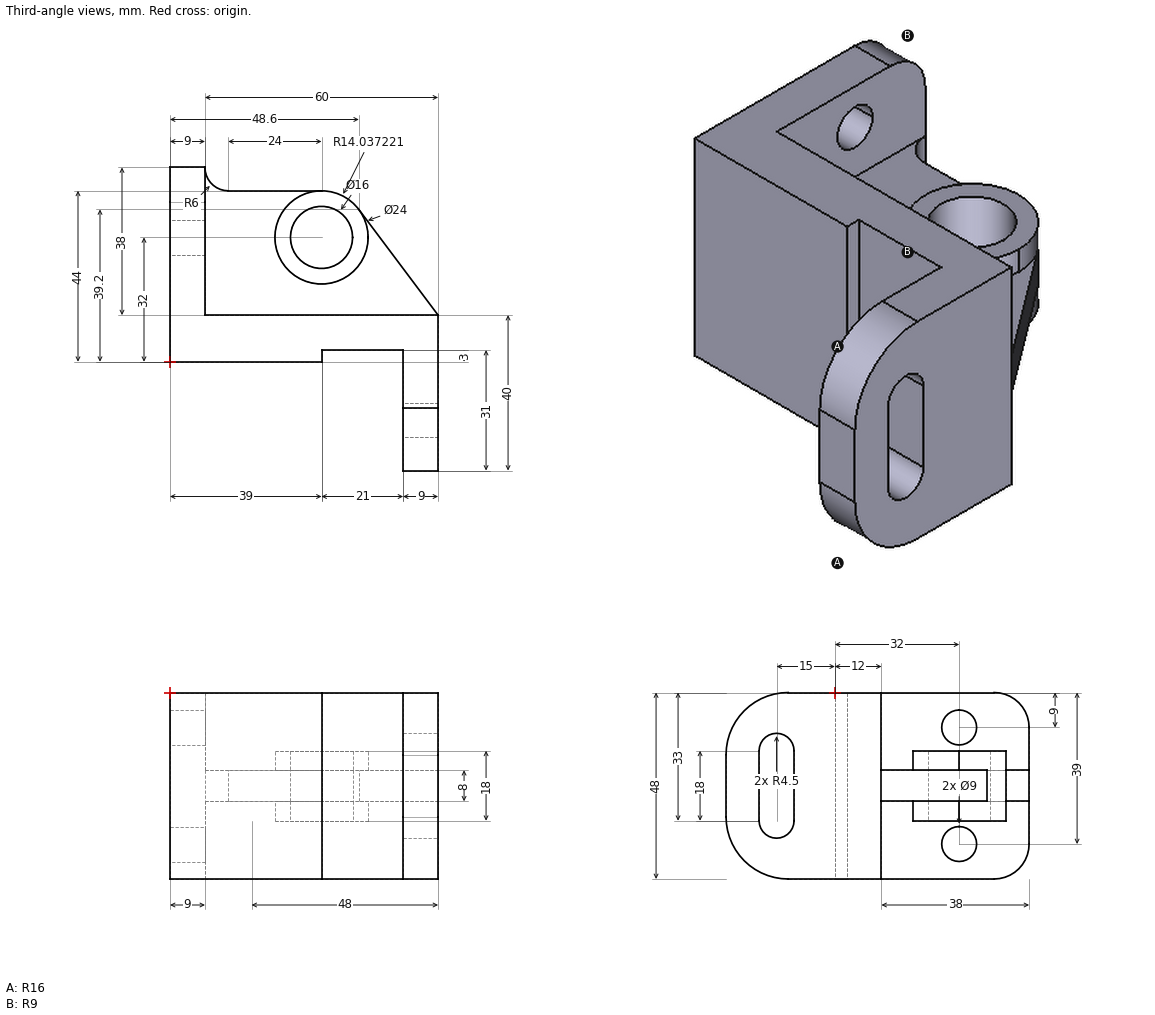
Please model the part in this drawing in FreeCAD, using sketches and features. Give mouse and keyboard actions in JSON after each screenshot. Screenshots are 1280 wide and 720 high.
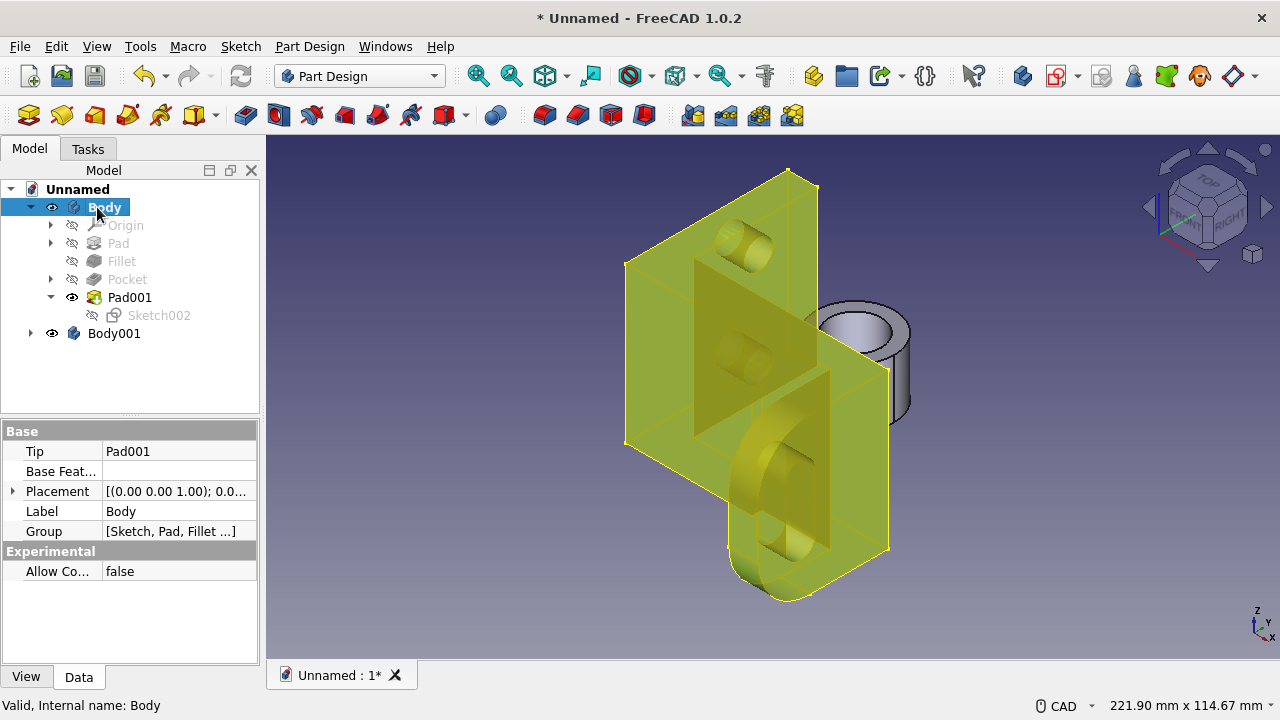
{"action": "left_click", "coordinate": [97, 207]}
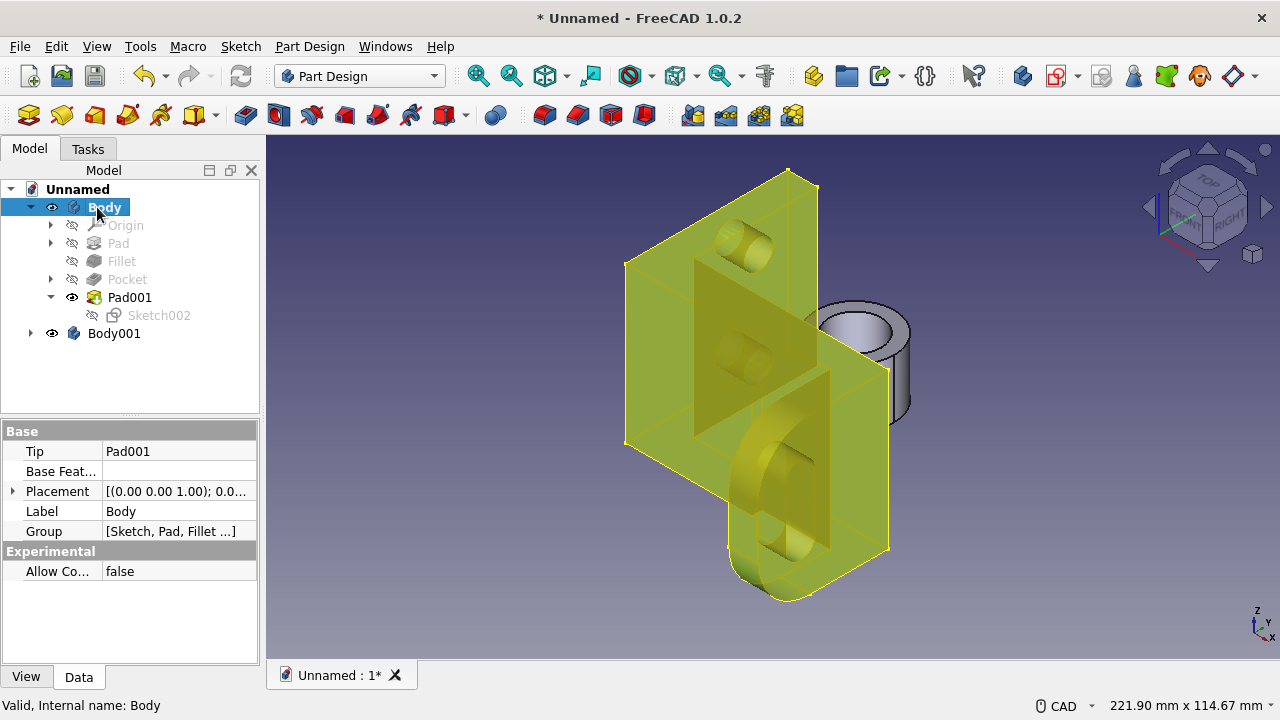
{"action": "left_click", "coordinate": [148, 571]}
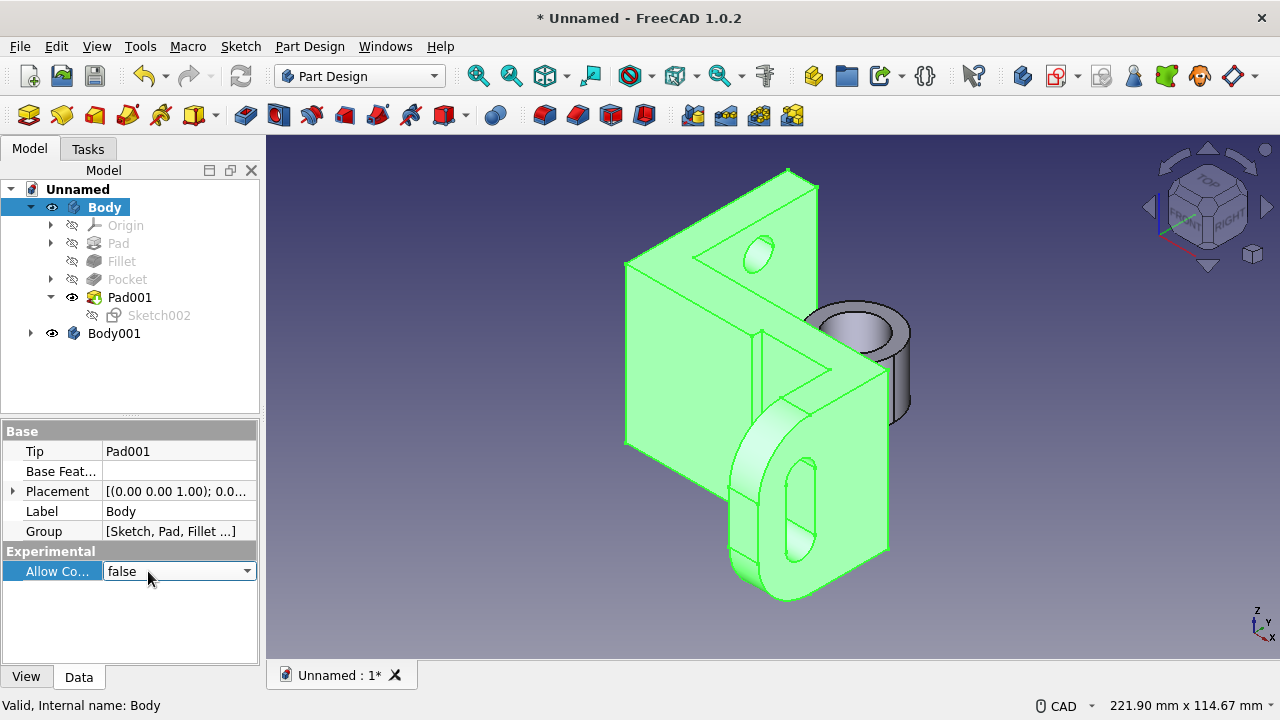
{"action": "left_click", "coordinate": [148, 571]}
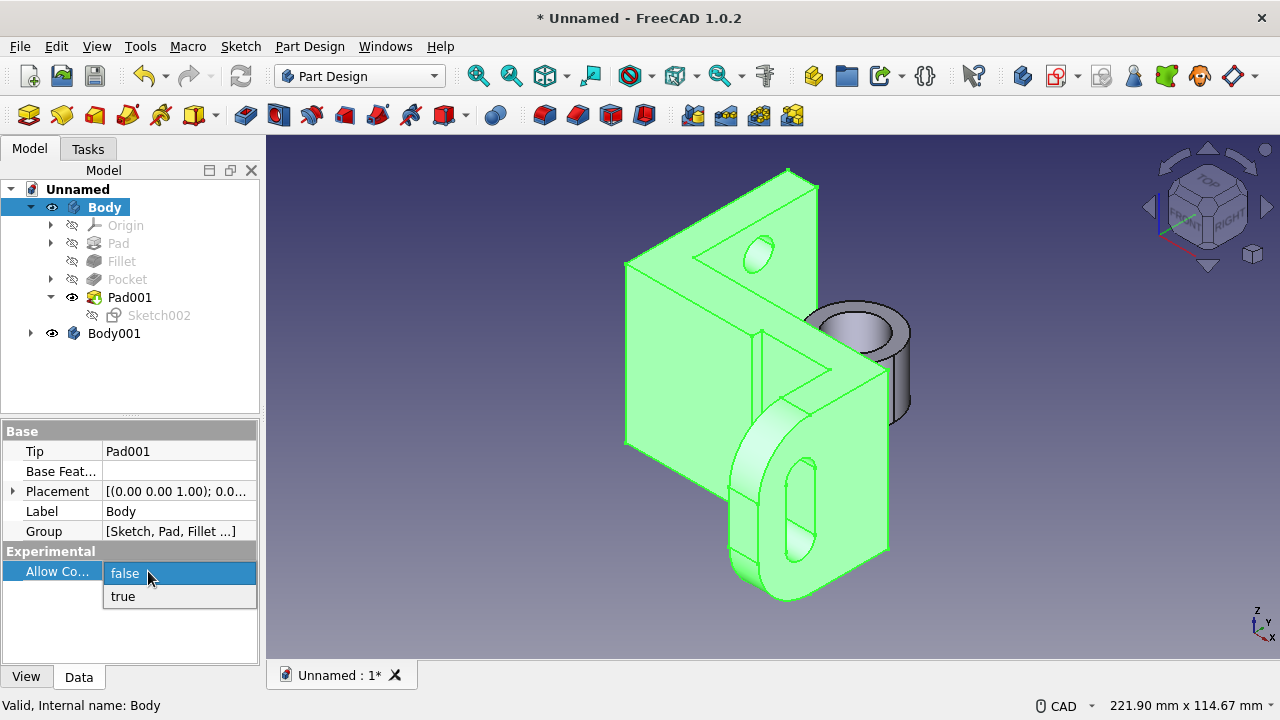
{"action": "left_click", "coordinate": [178, 596]}
{"action": "key", "text": "Return"}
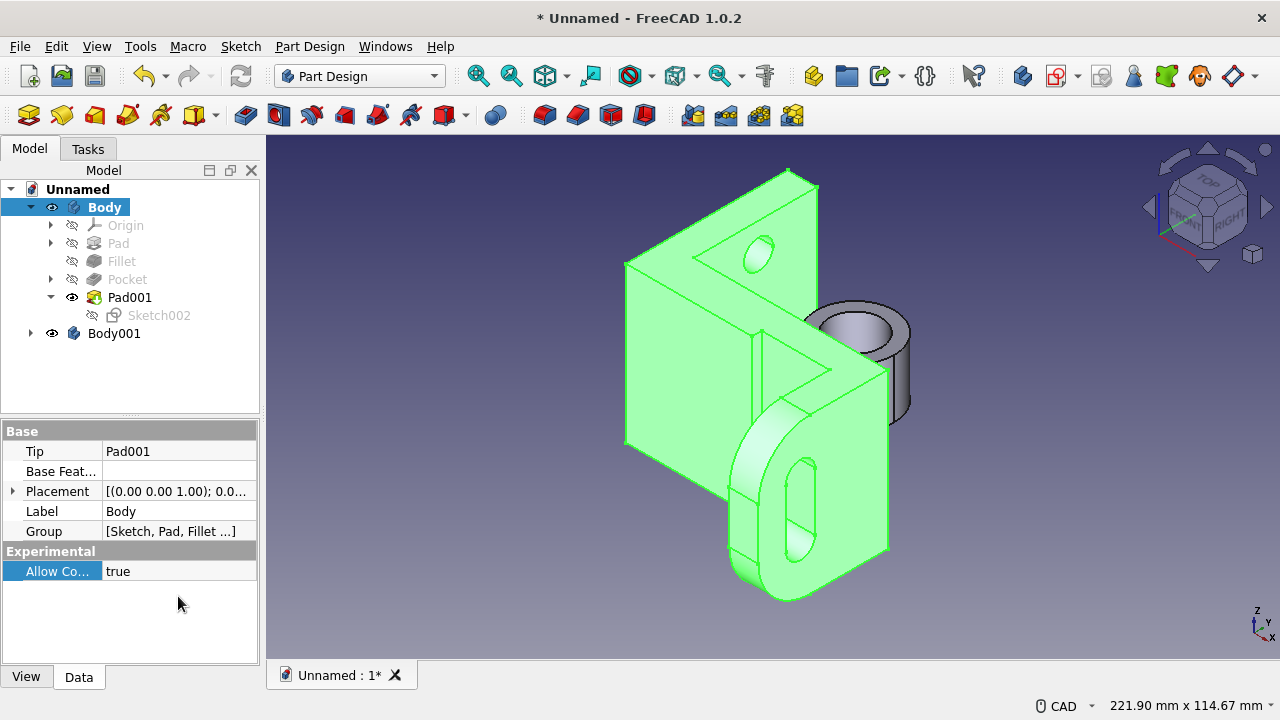
{"action": "left_click", "coordinate": [97, 333]}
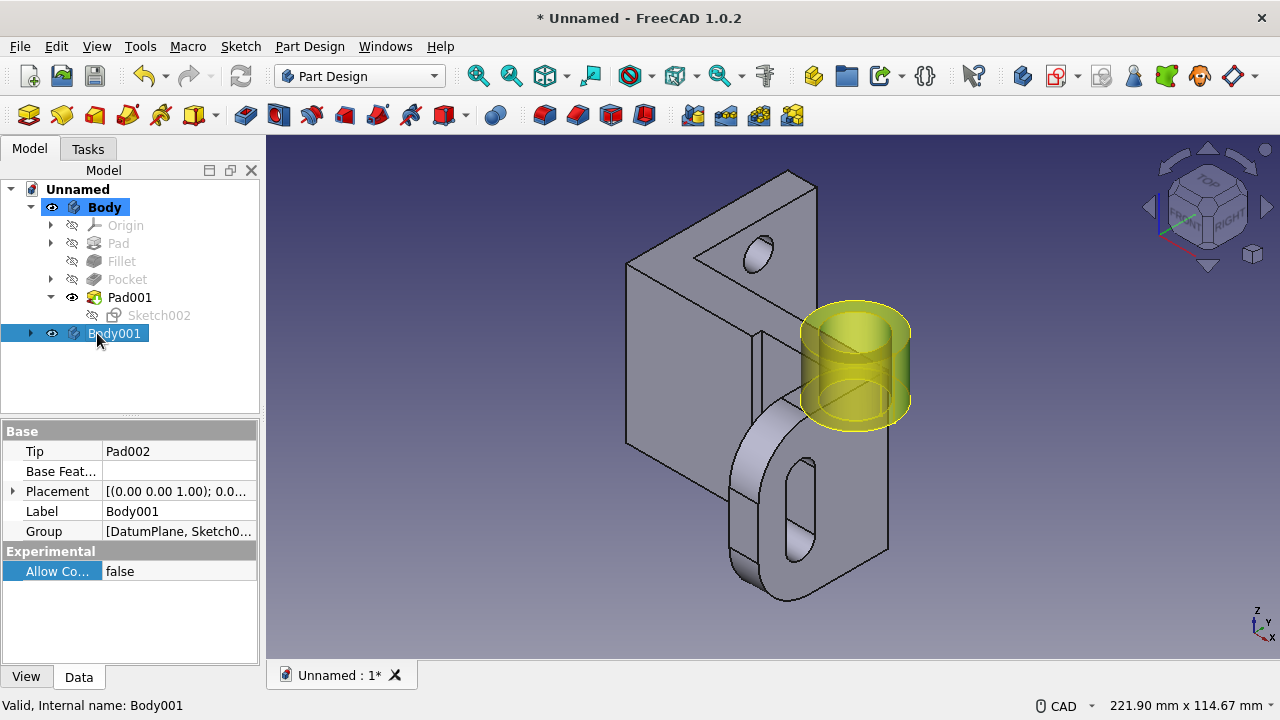
{"action": "left_click", "coordinate": [496, 116]}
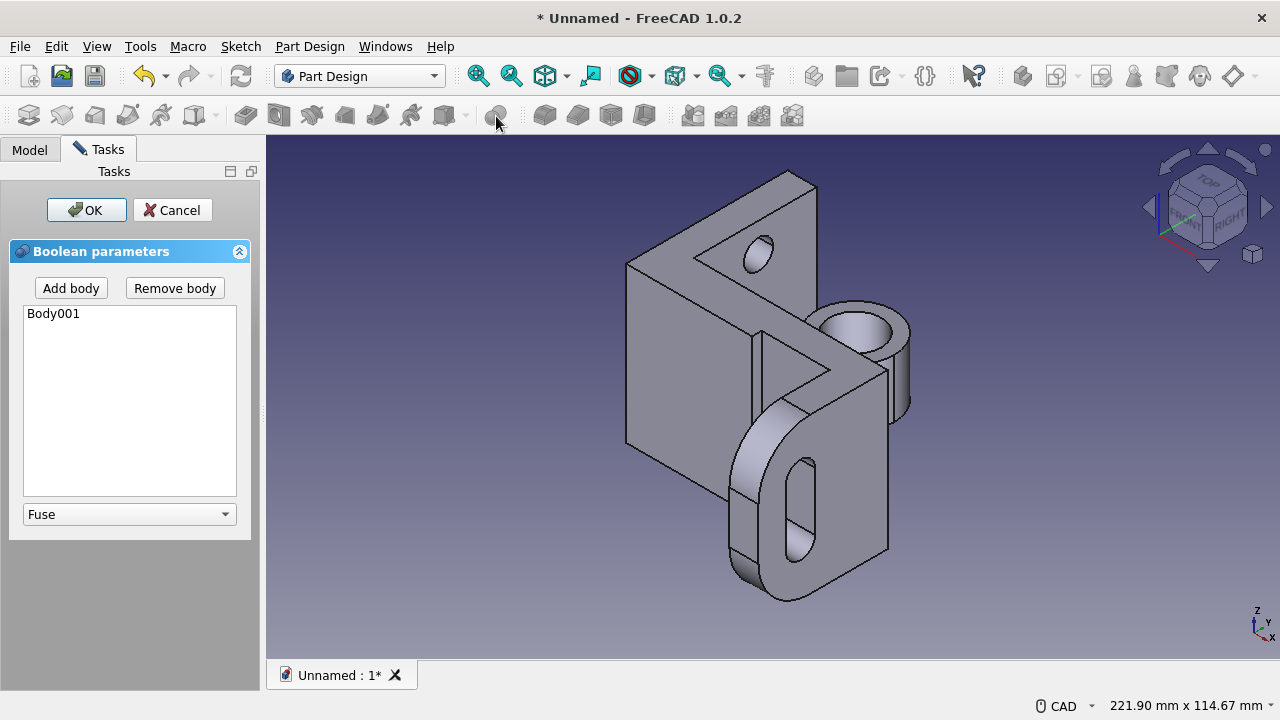
{"action": "left_click", "coordinate": [87, 210]}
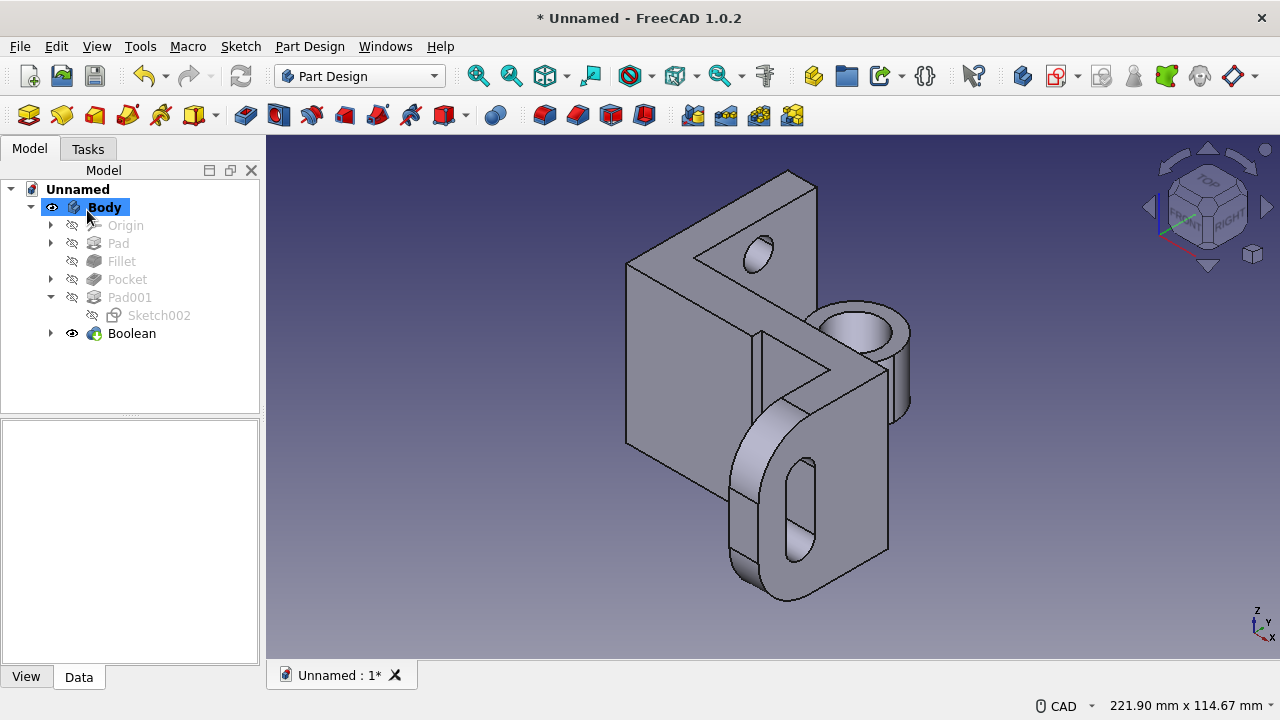
{"action": "left_click", "coordinate": [51, 225]}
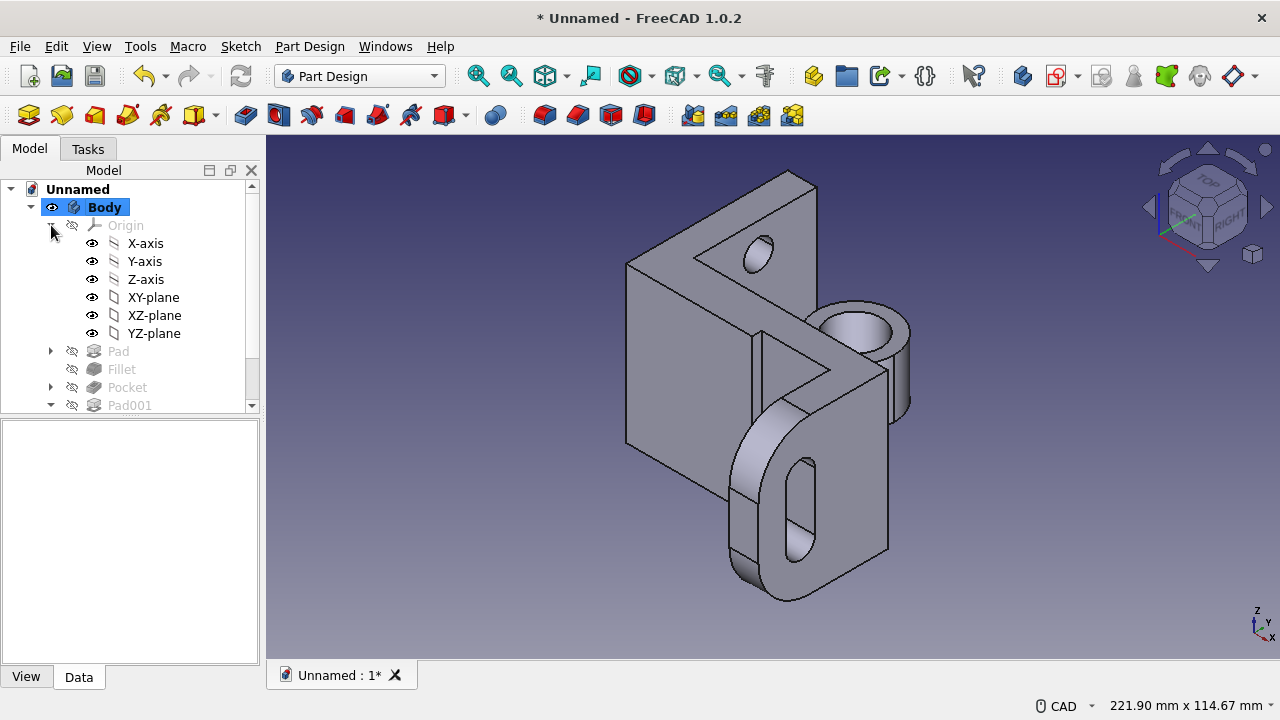
{"action": "left_click", "coordinate": [137, 297]}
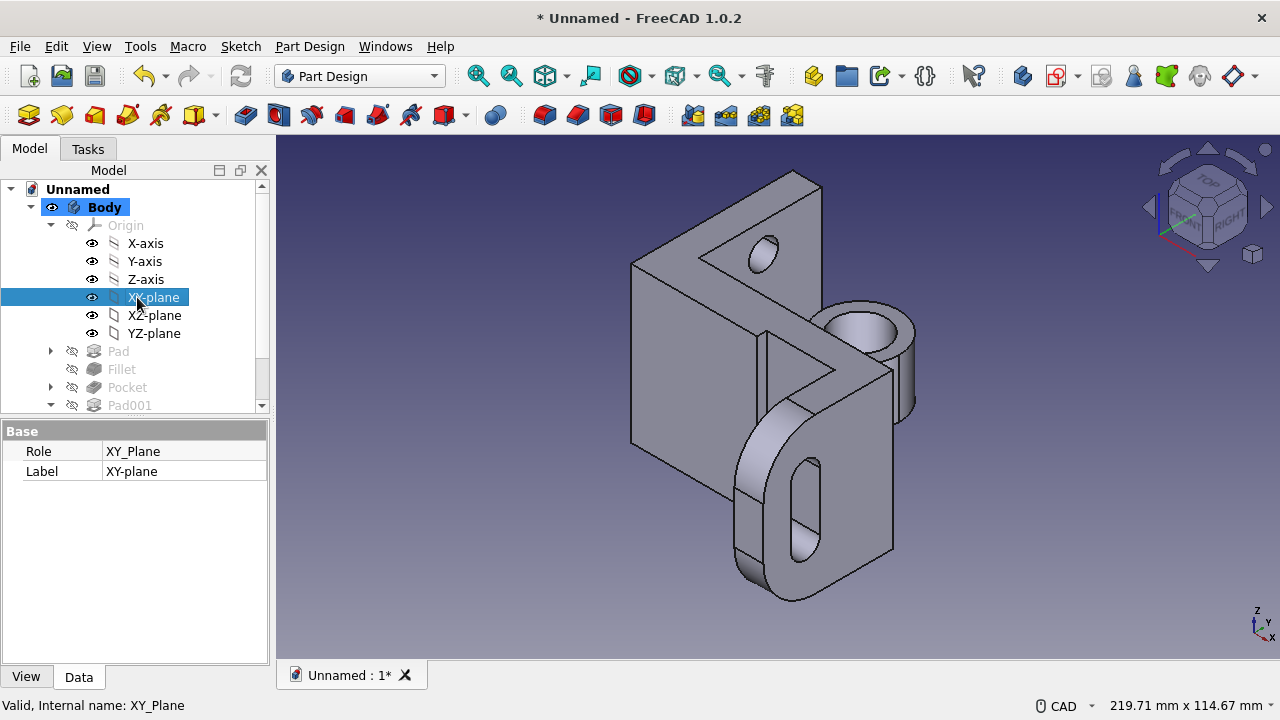
{"action": "left_click", "coordinate": [1232, 76]}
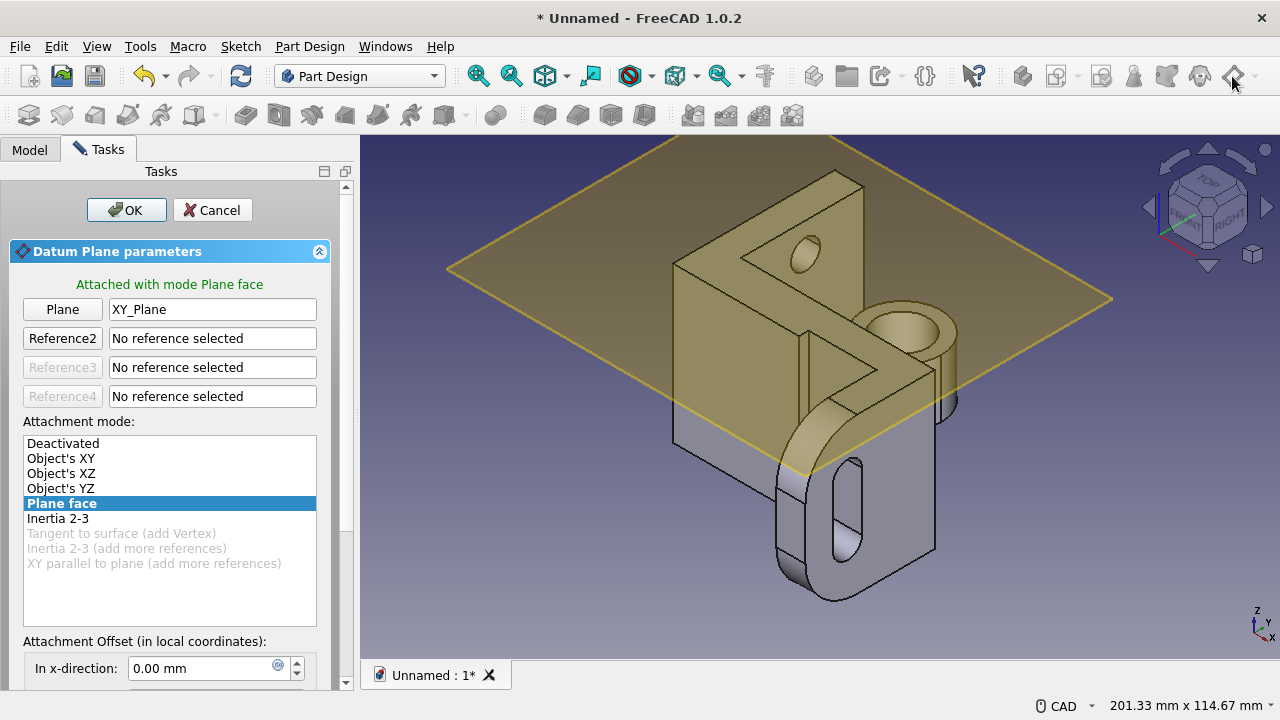
{"action": "scroll", "coordinate": [346, 436], "scroll_direction": "down", "scroll_amount": 2}